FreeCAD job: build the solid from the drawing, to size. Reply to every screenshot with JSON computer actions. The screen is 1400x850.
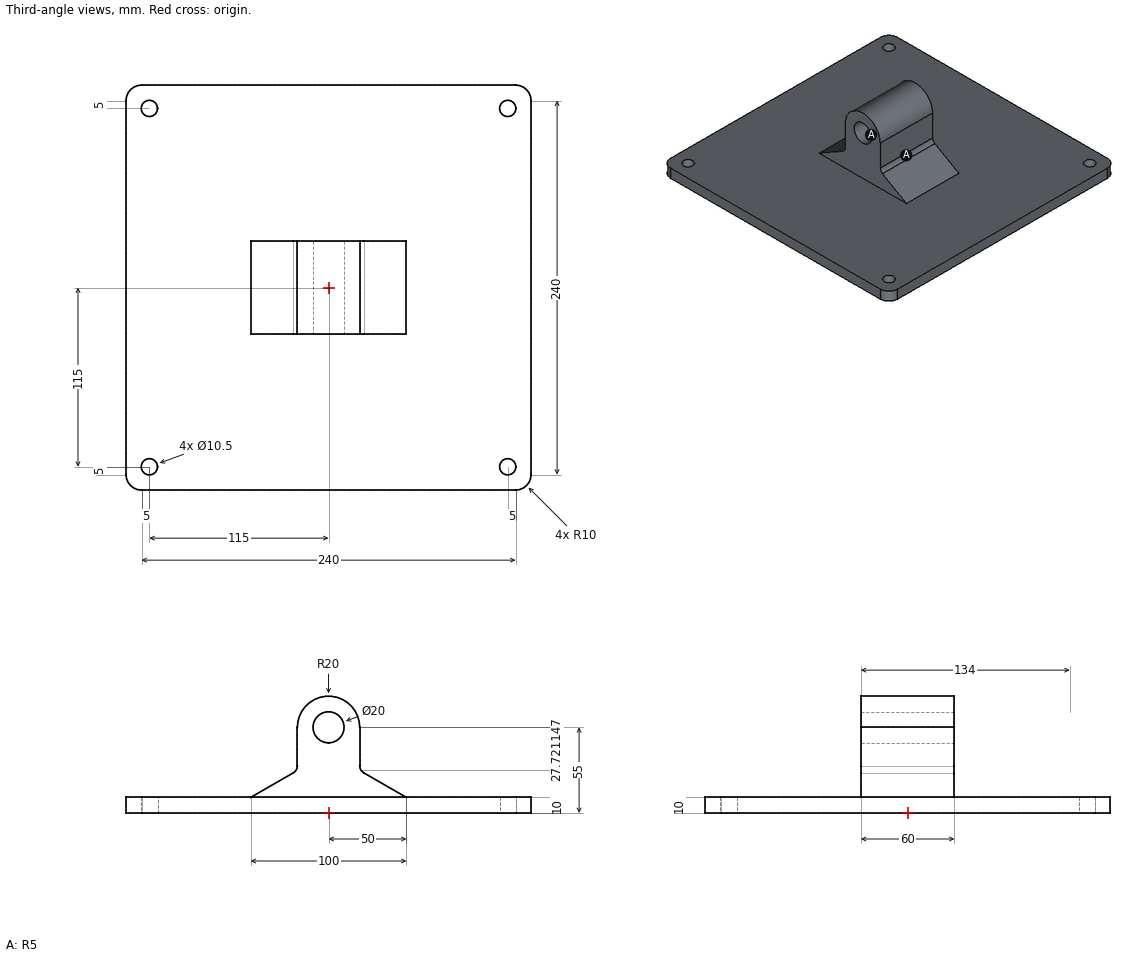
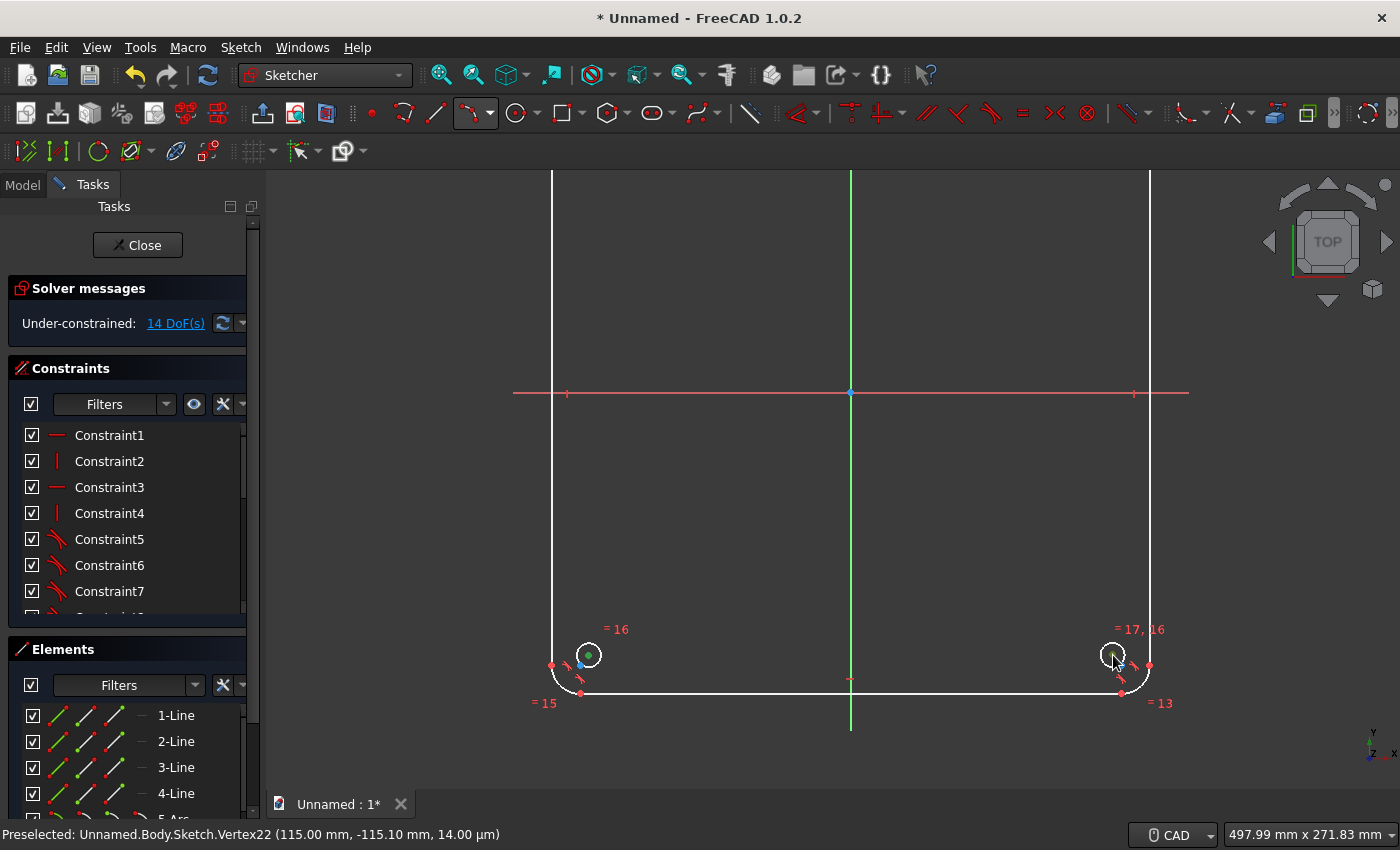
{"action": "key", "text": "h"}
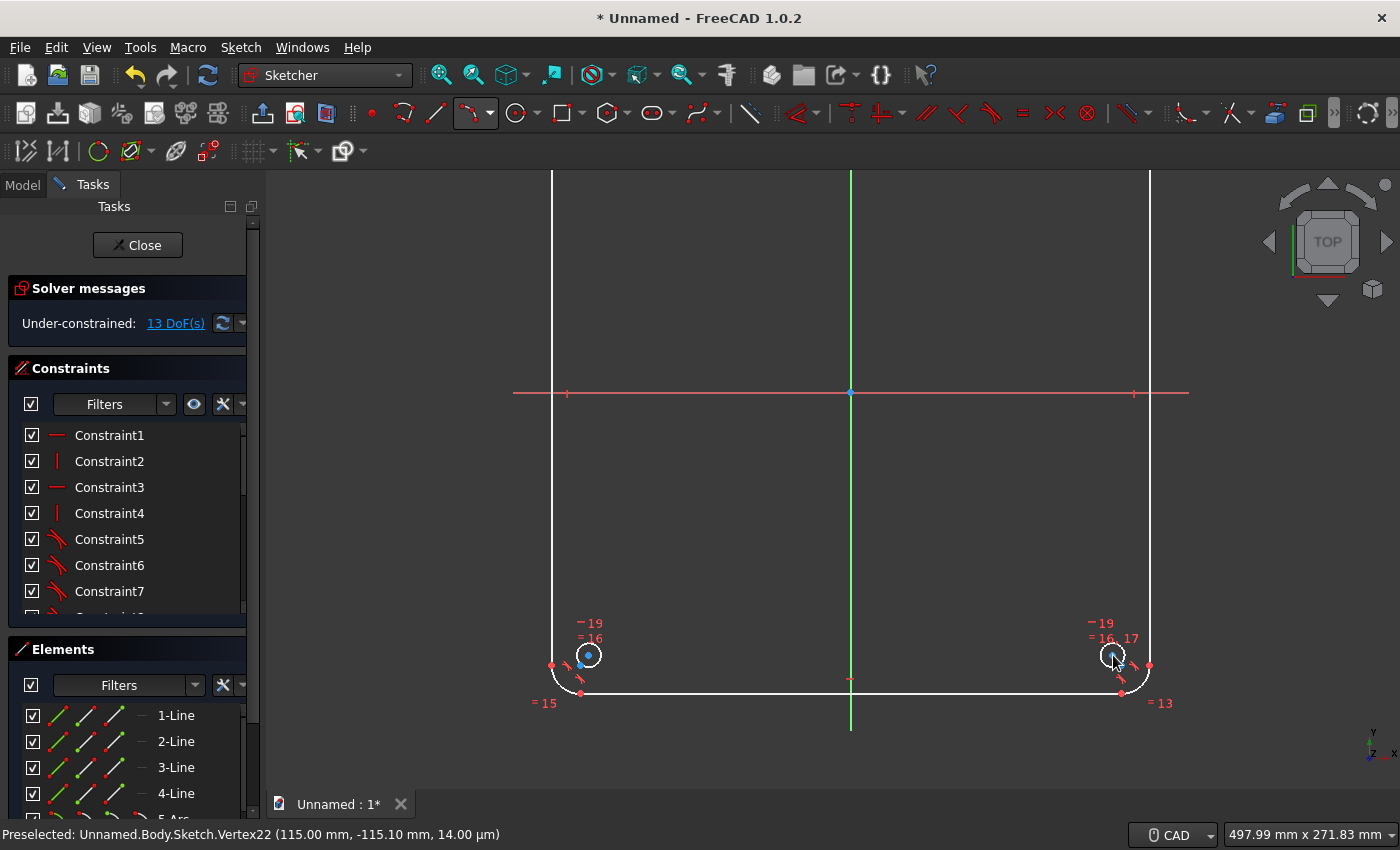
{"action": "left_click", "coordinate": [589, 655]}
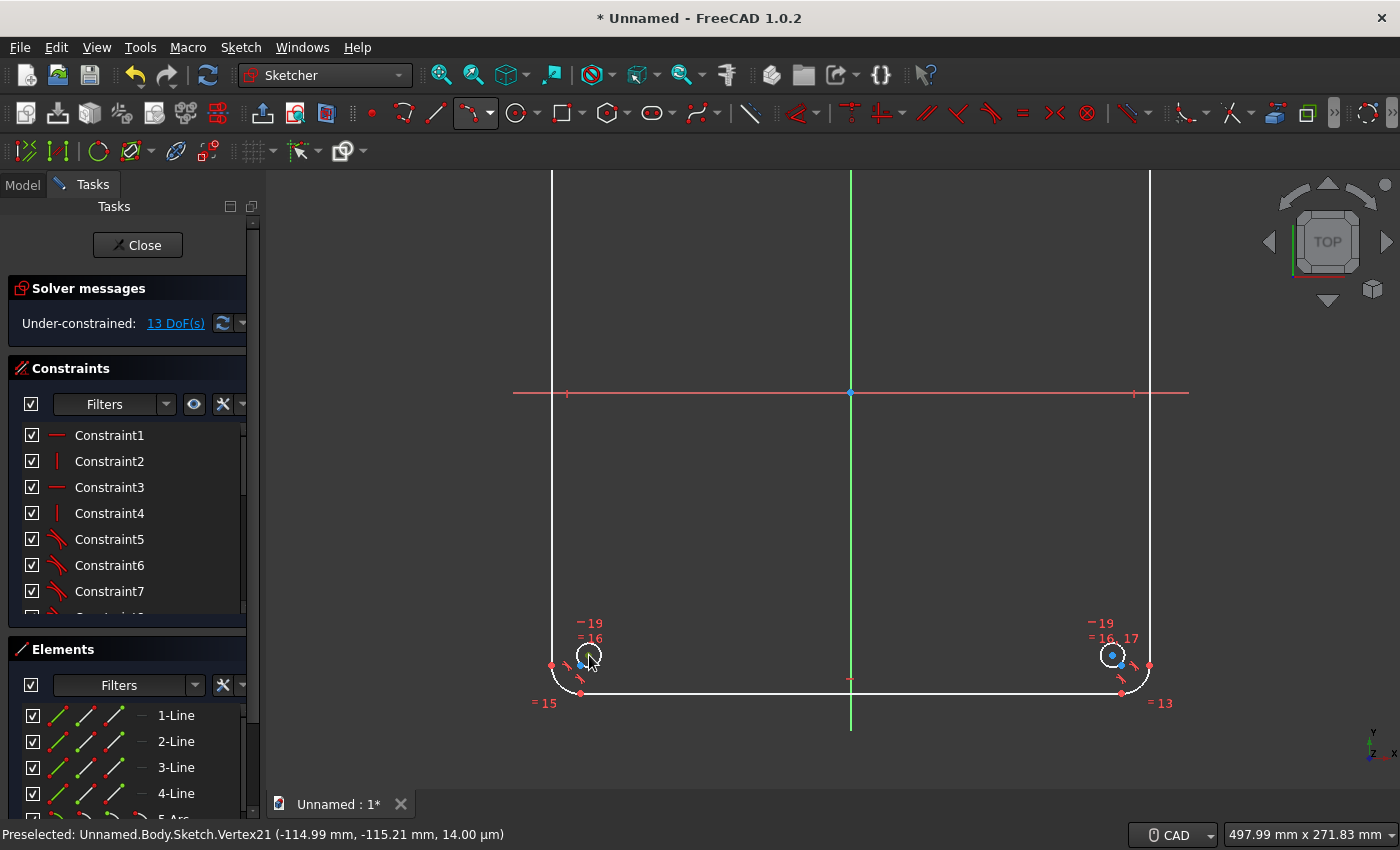
{"action": "scroll", "coordinate": [589, 656], "scroll_direction": "down", "scroll_amount": 2}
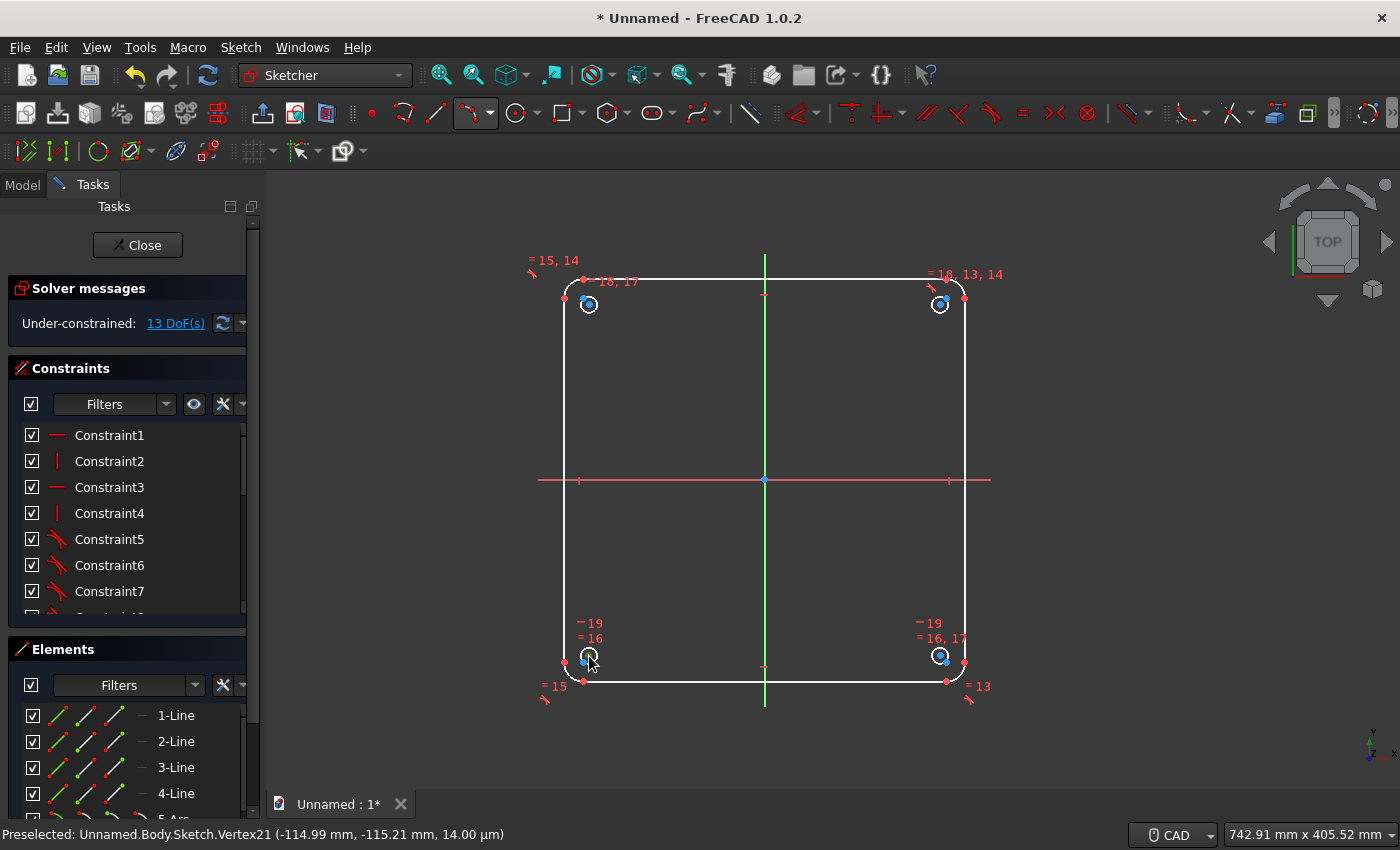
{"action": "scroll", "coordinate": [589, 305], "scroll_direction": "up", "scroll_amount": 2}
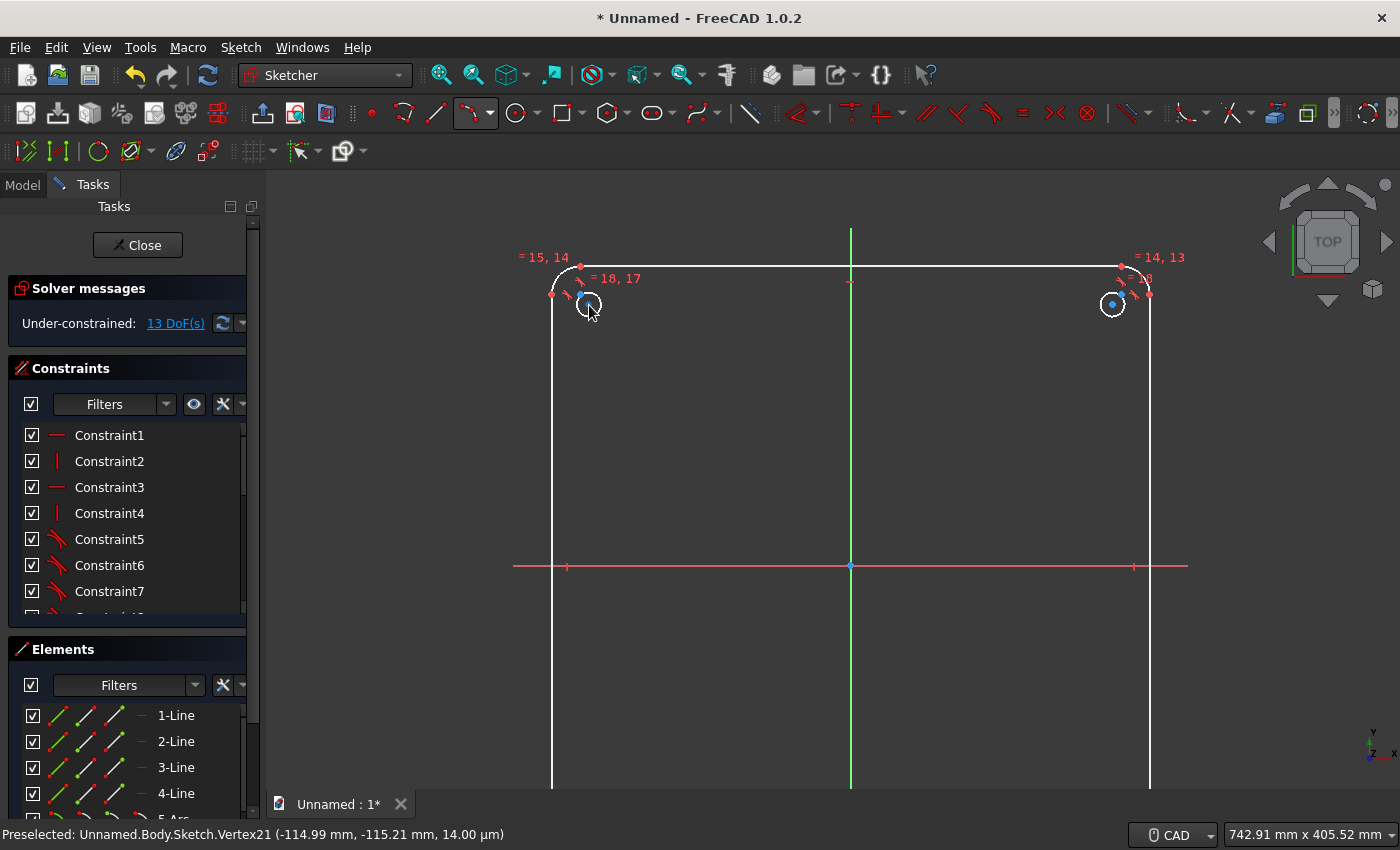
{"action": "left_click", "coordinate": [589, 305]}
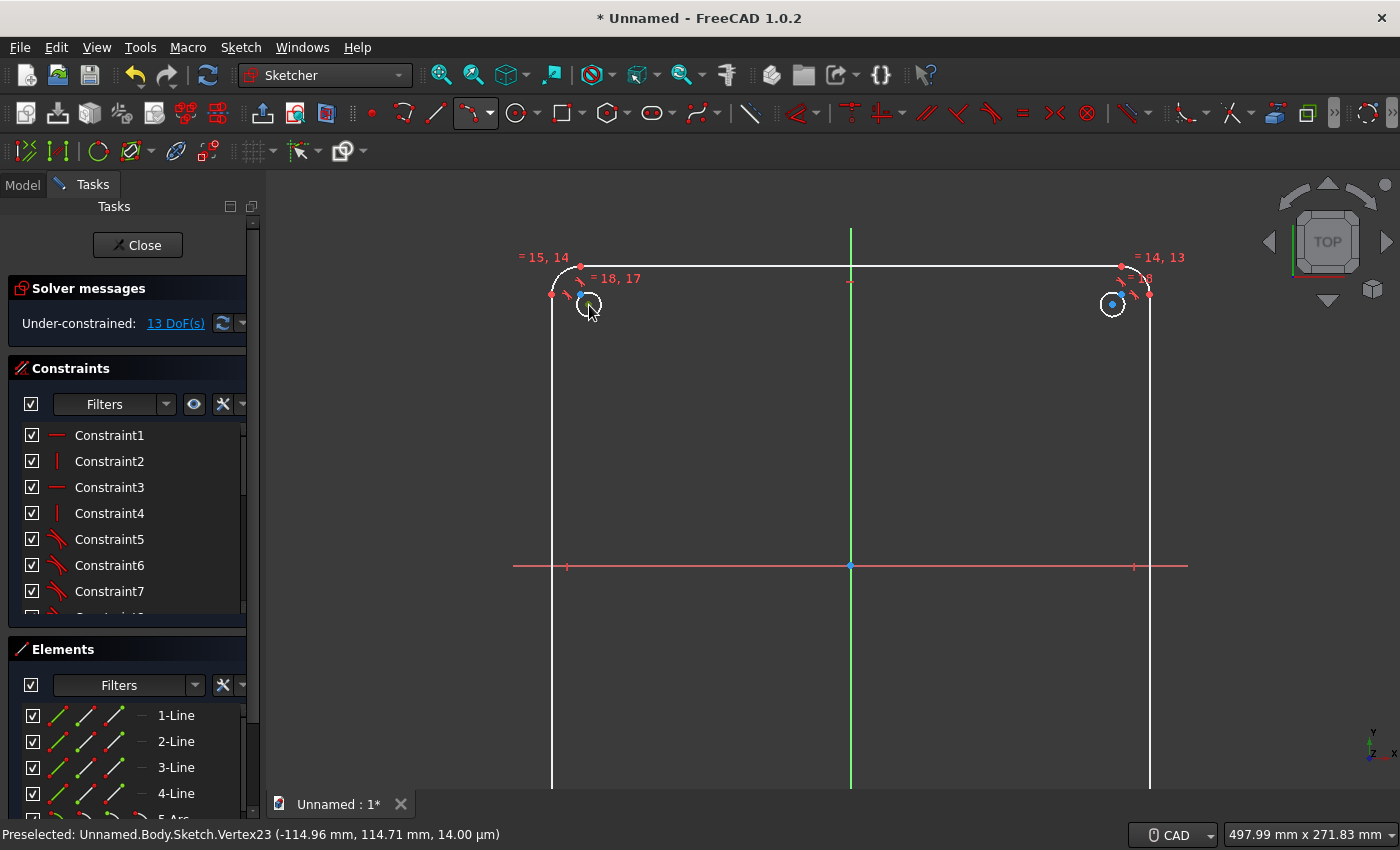
{"action": "left_click", "coordinate": [904, 114]}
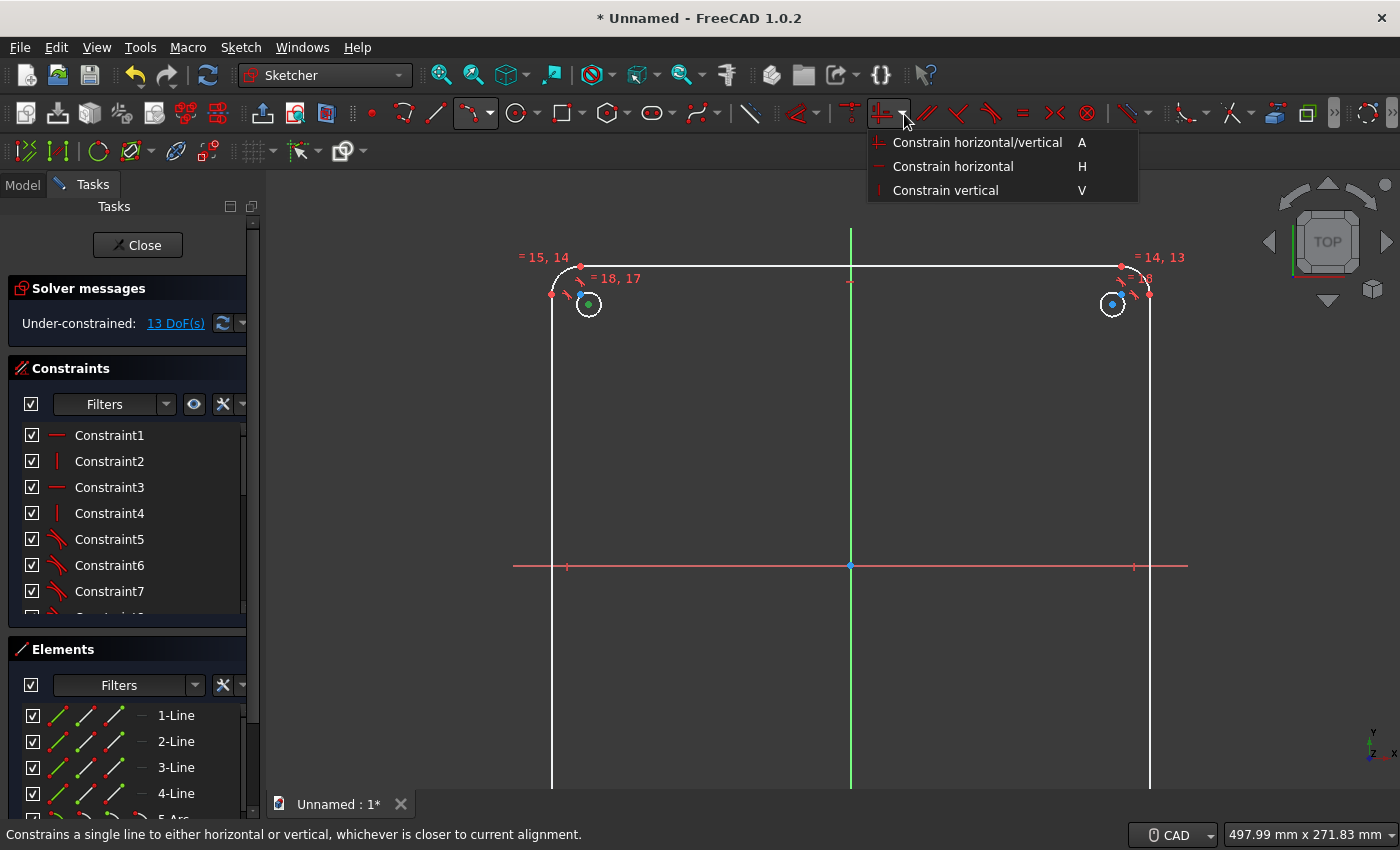
{"action": "left_click", "coordinate": [1003, 190]}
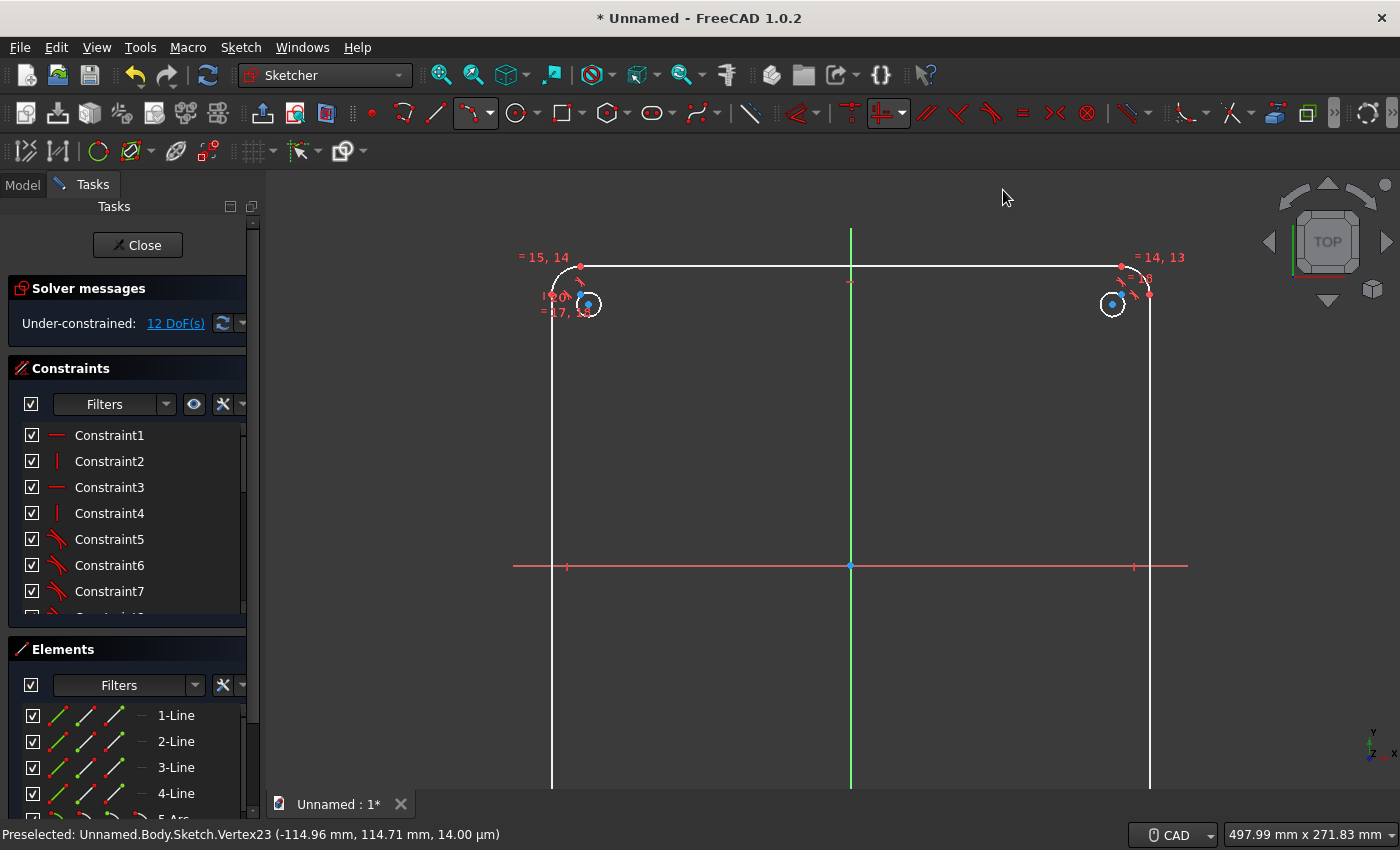
{"action": "scroll", "coordinate": [589, 304], "scroll_direction": "down", "scroll_amount": 2}